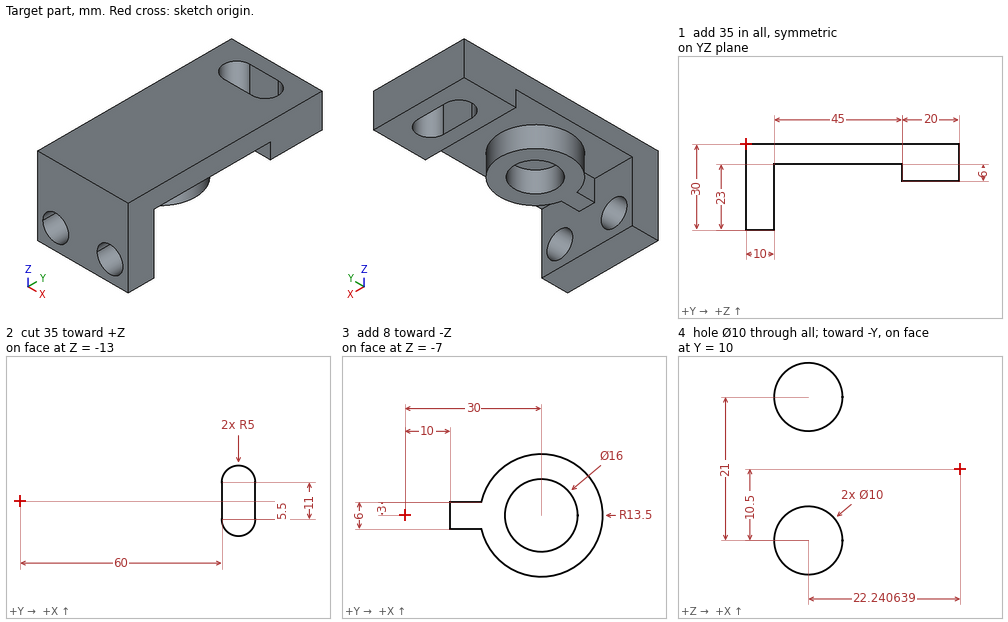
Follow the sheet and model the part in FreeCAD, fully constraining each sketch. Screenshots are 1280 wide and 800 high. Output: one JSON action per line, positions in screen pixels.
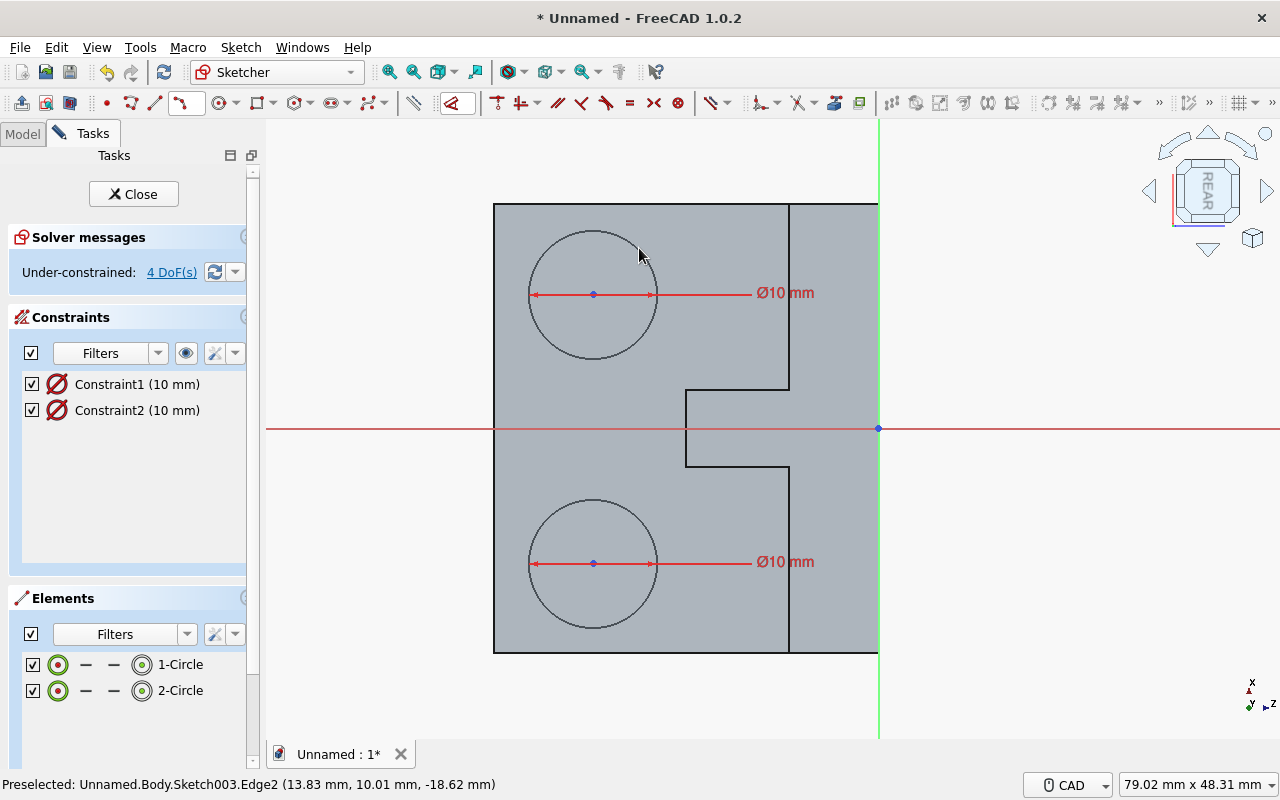
{"action": "left_click", "coordinate": [593, 564]}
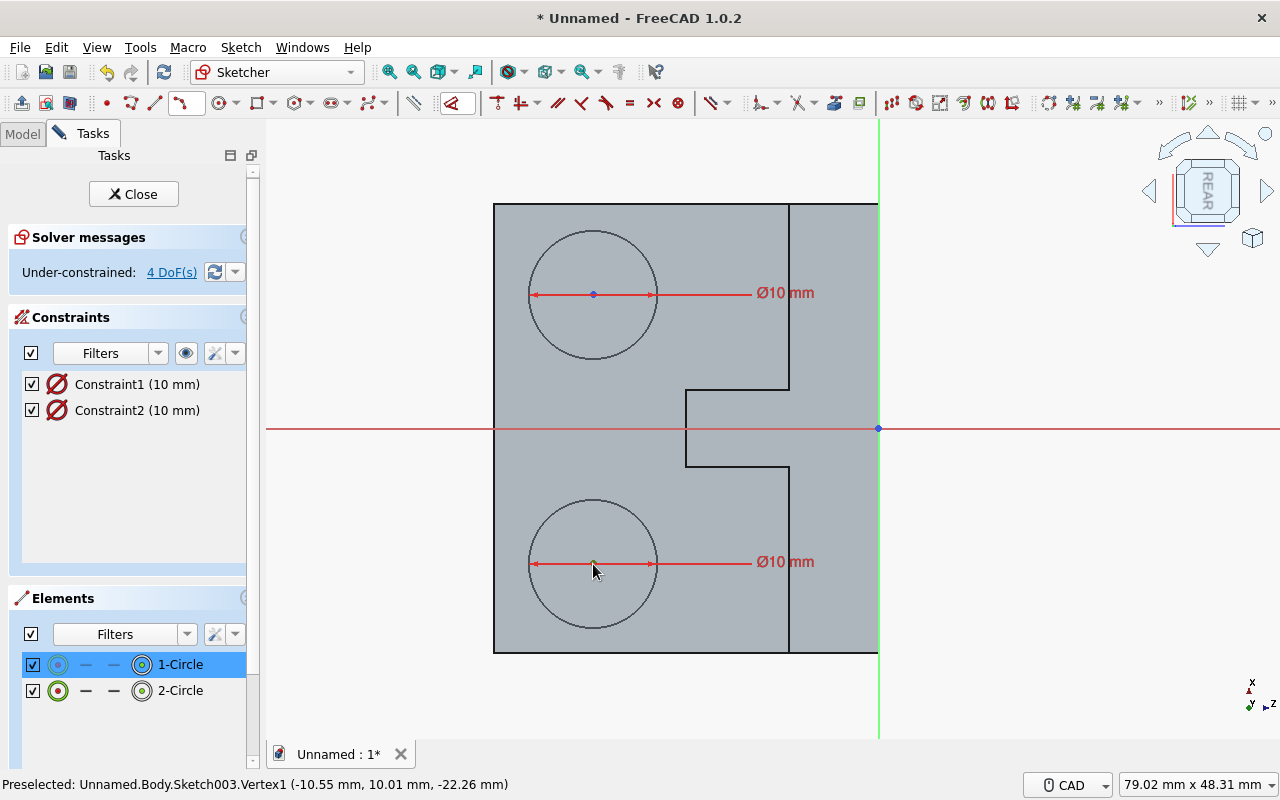
{"action": "left_click", "coordinate": [593, 295]}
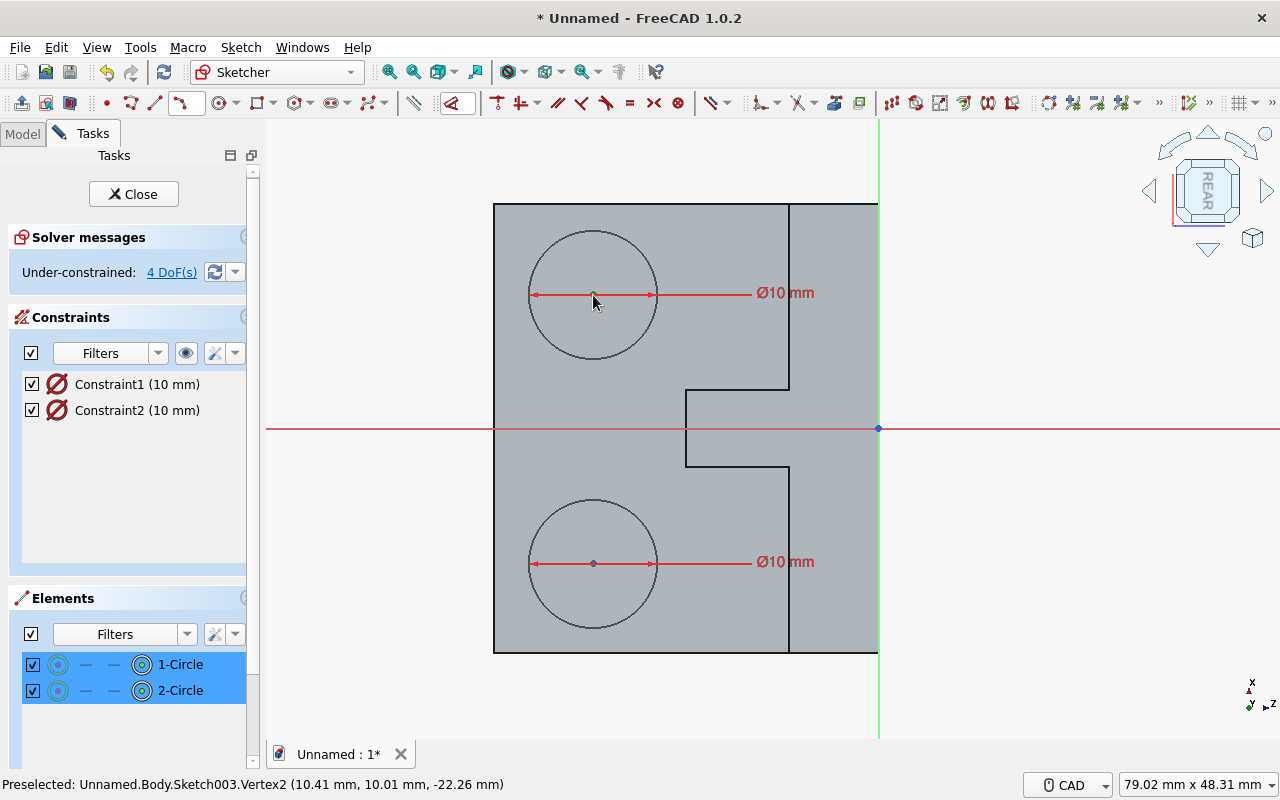
{"action": "left_click", "coordinate": [540, 104]}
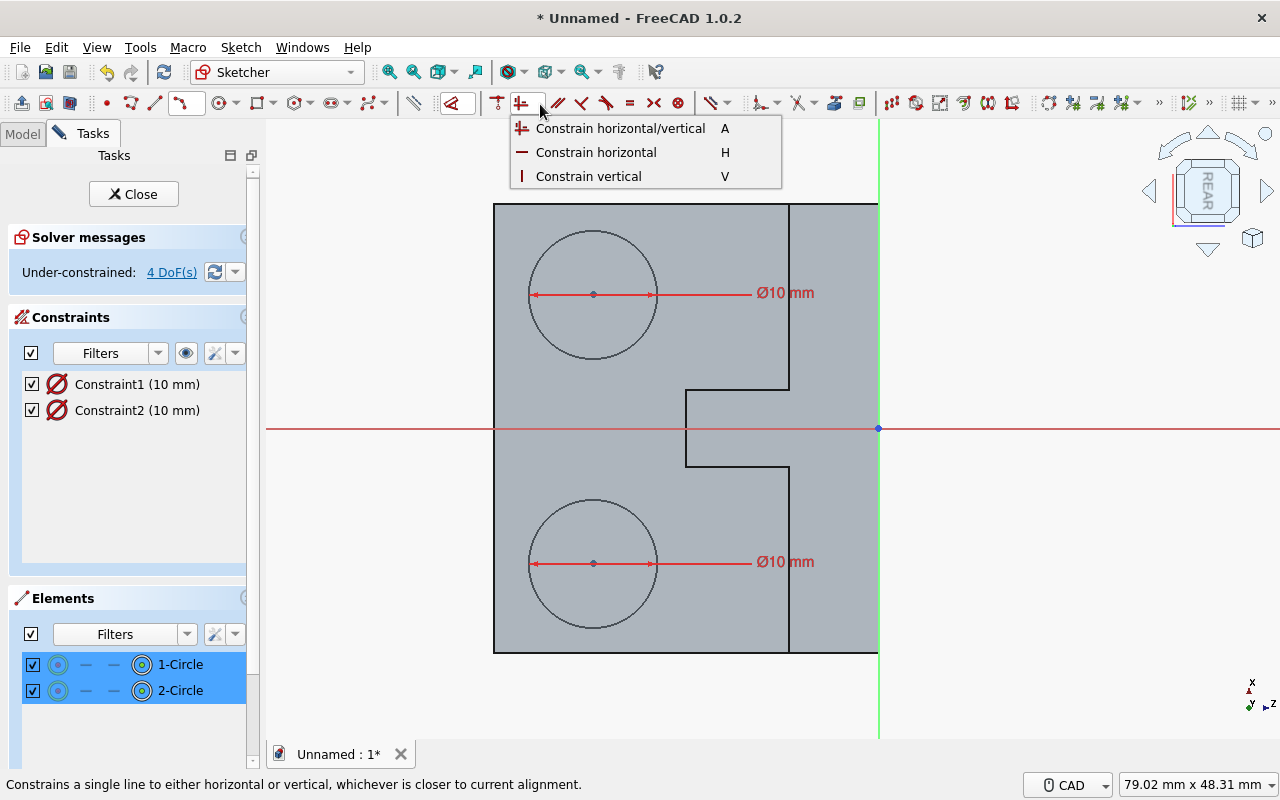
{"action": "left_click", "coordinate": [646, 176]}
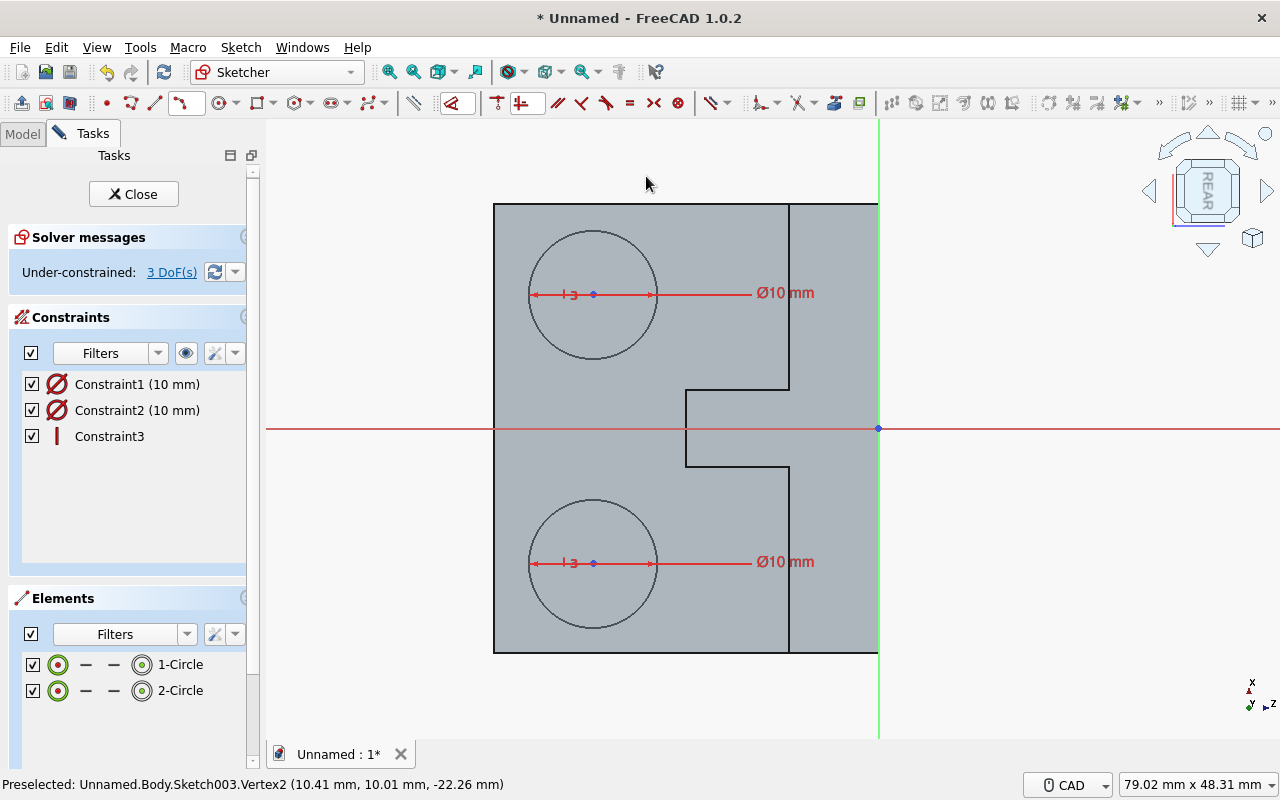
{"action": "left_click", "coordinate": [593, 564]}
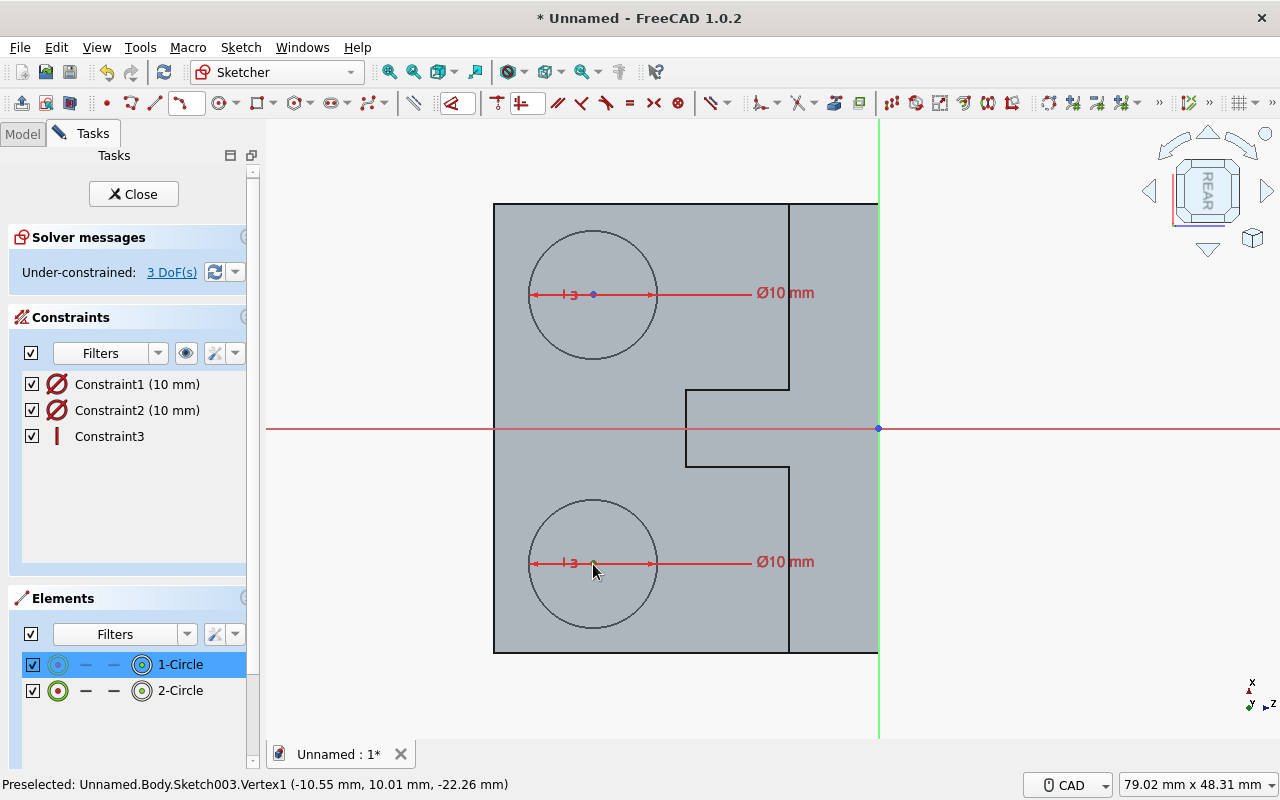
{"action": "left_click", "coordinate": [593, 295]}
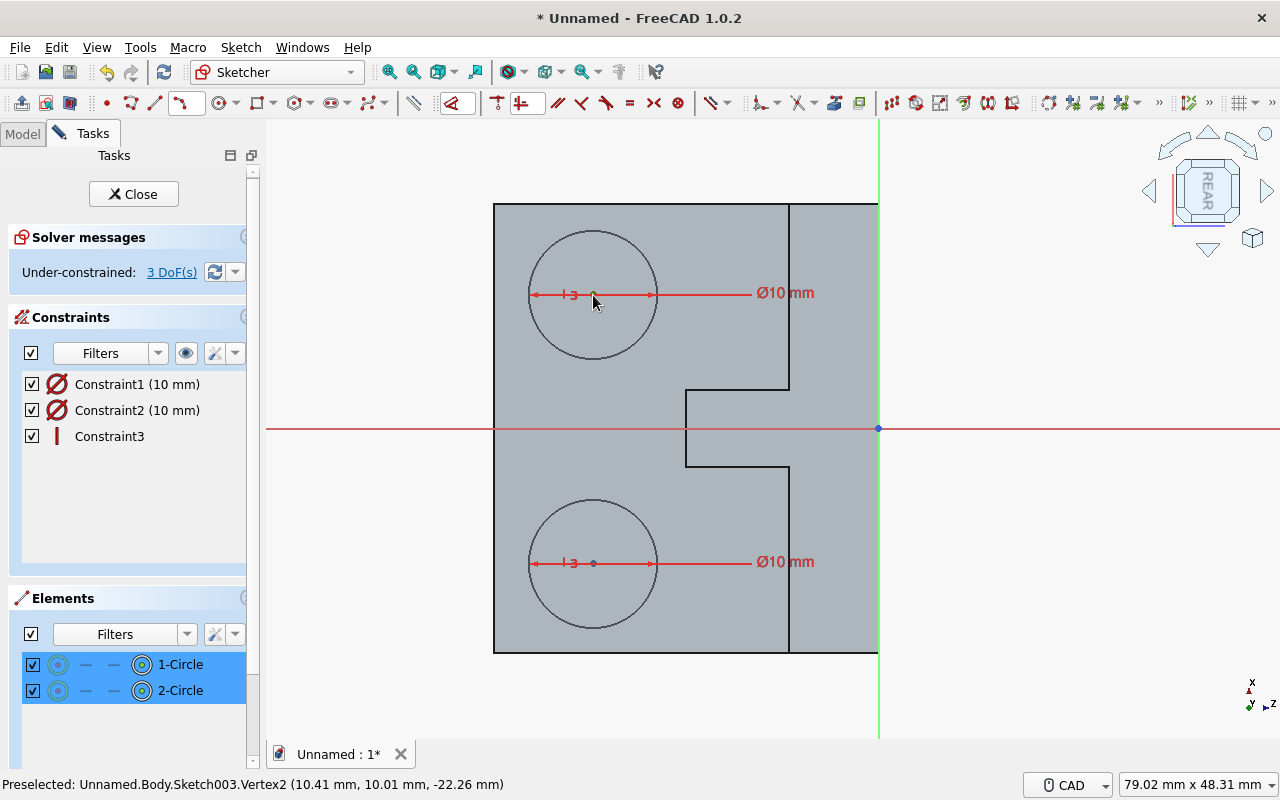
{"action": "key", "text": "i"}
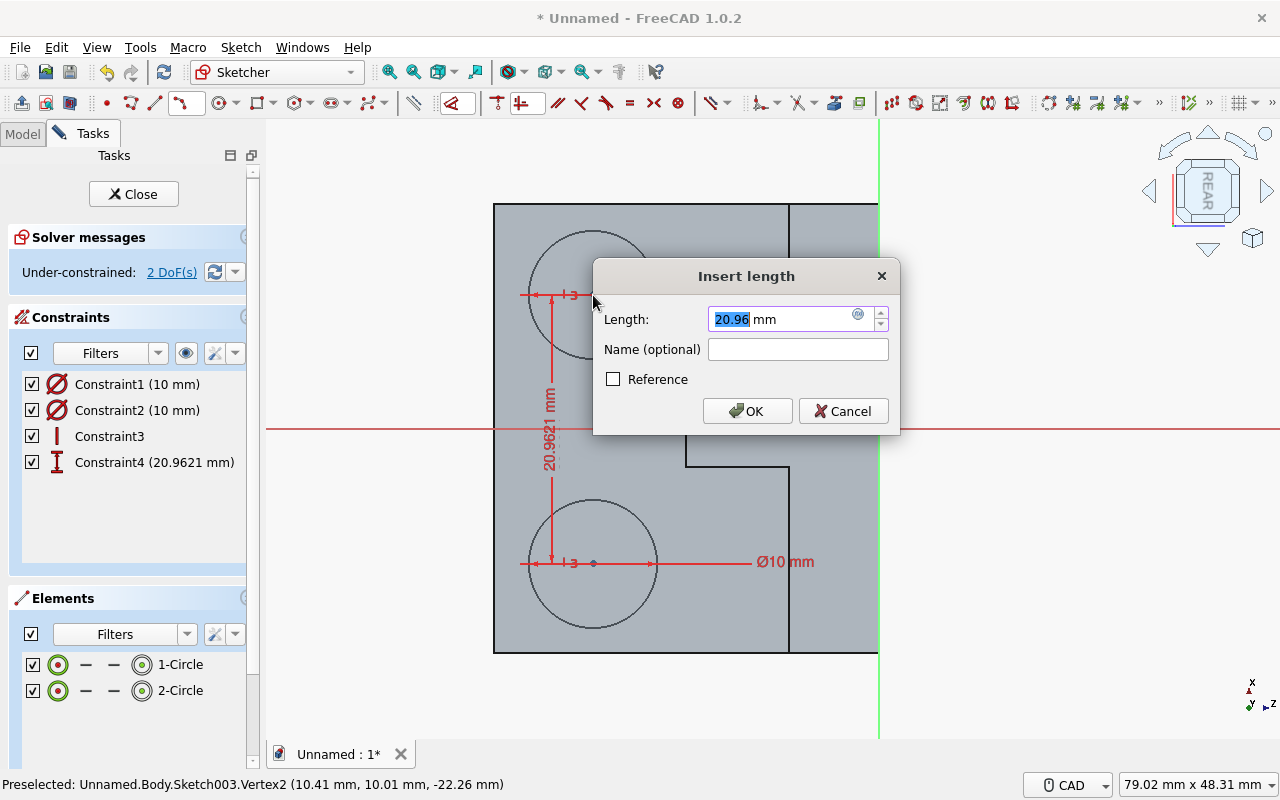
{"action": "type", "text": "21"}
{"action": "key", "text": "Return"}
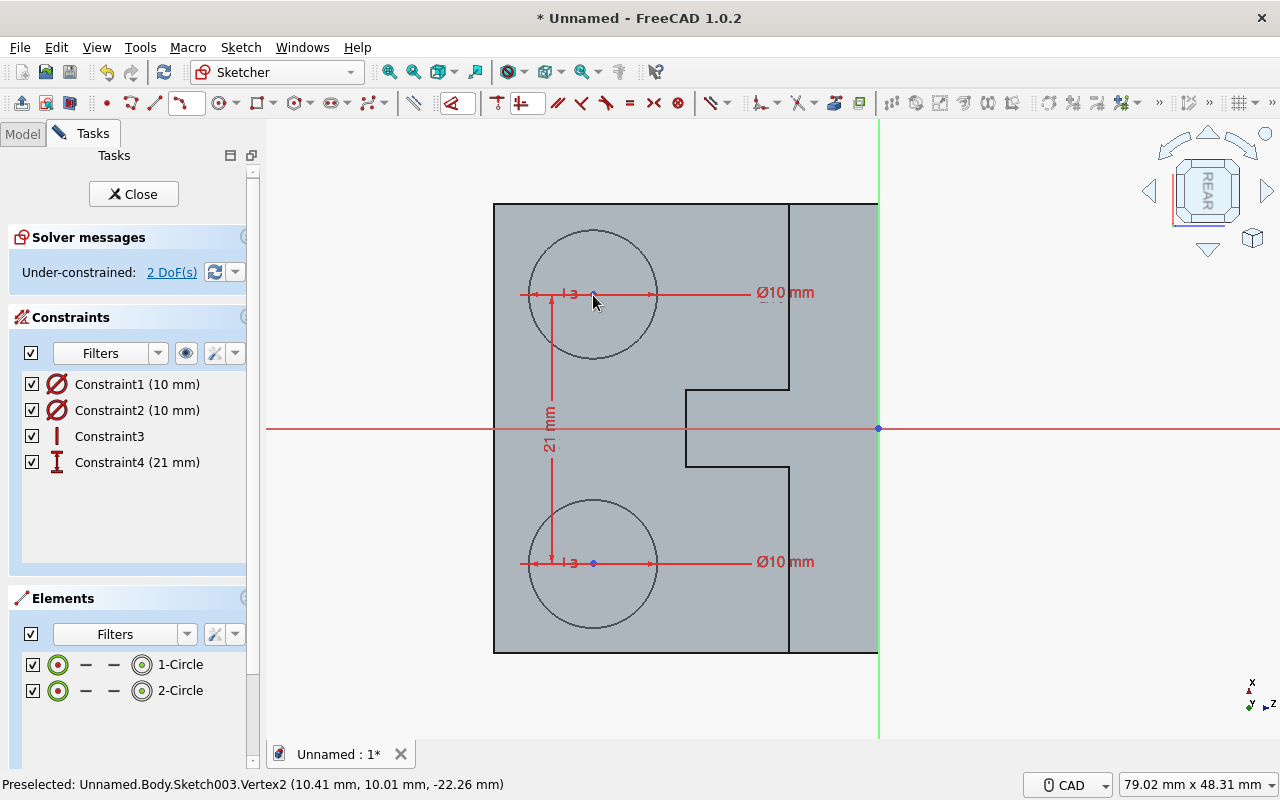
{"action": "left_click", "coordinate": [593, 564]}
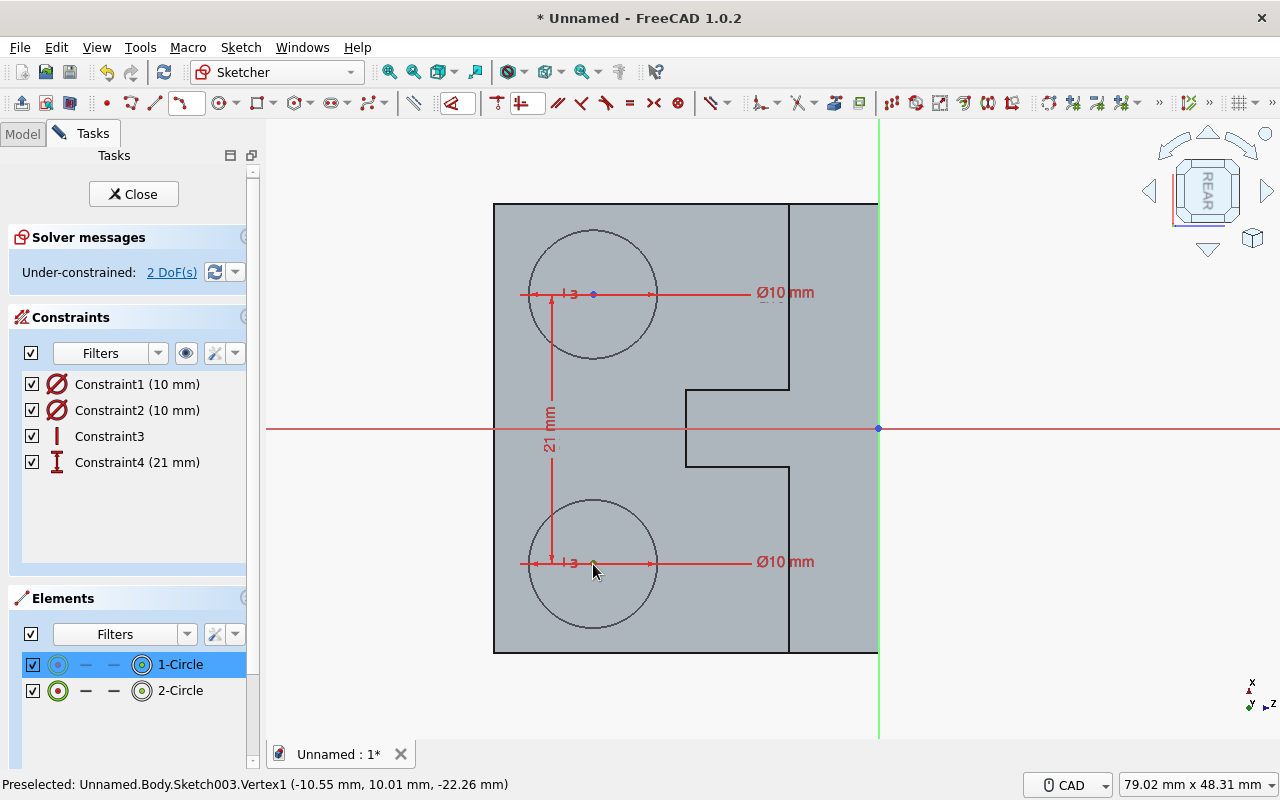
{"action": "key", "text": "i"}